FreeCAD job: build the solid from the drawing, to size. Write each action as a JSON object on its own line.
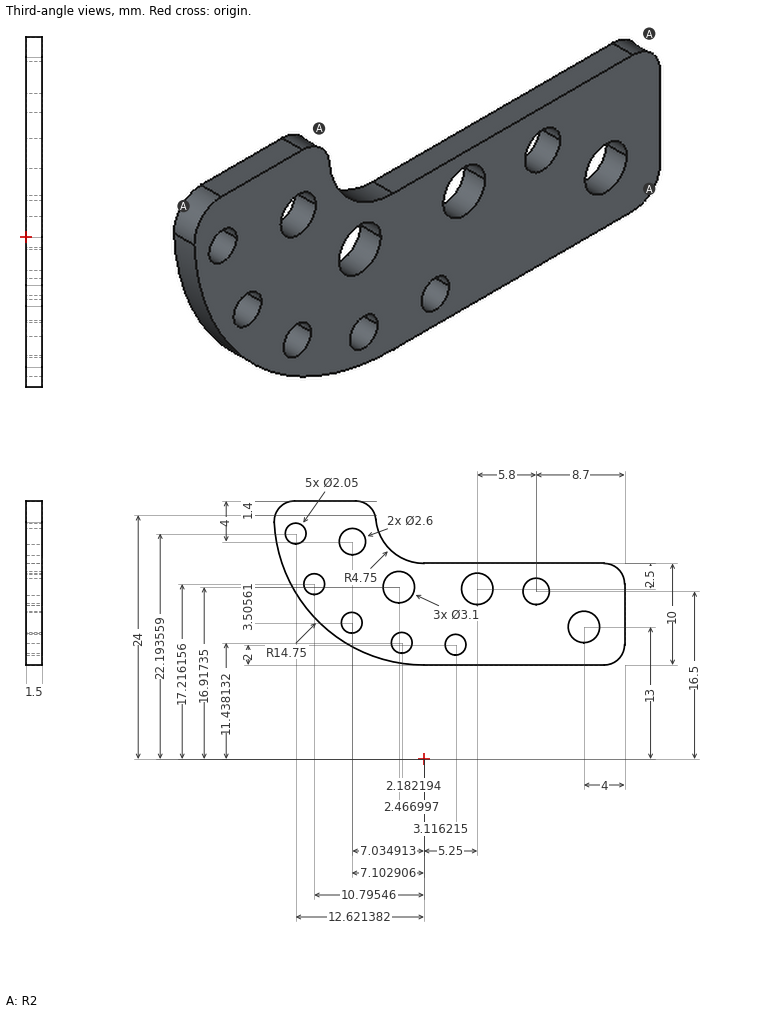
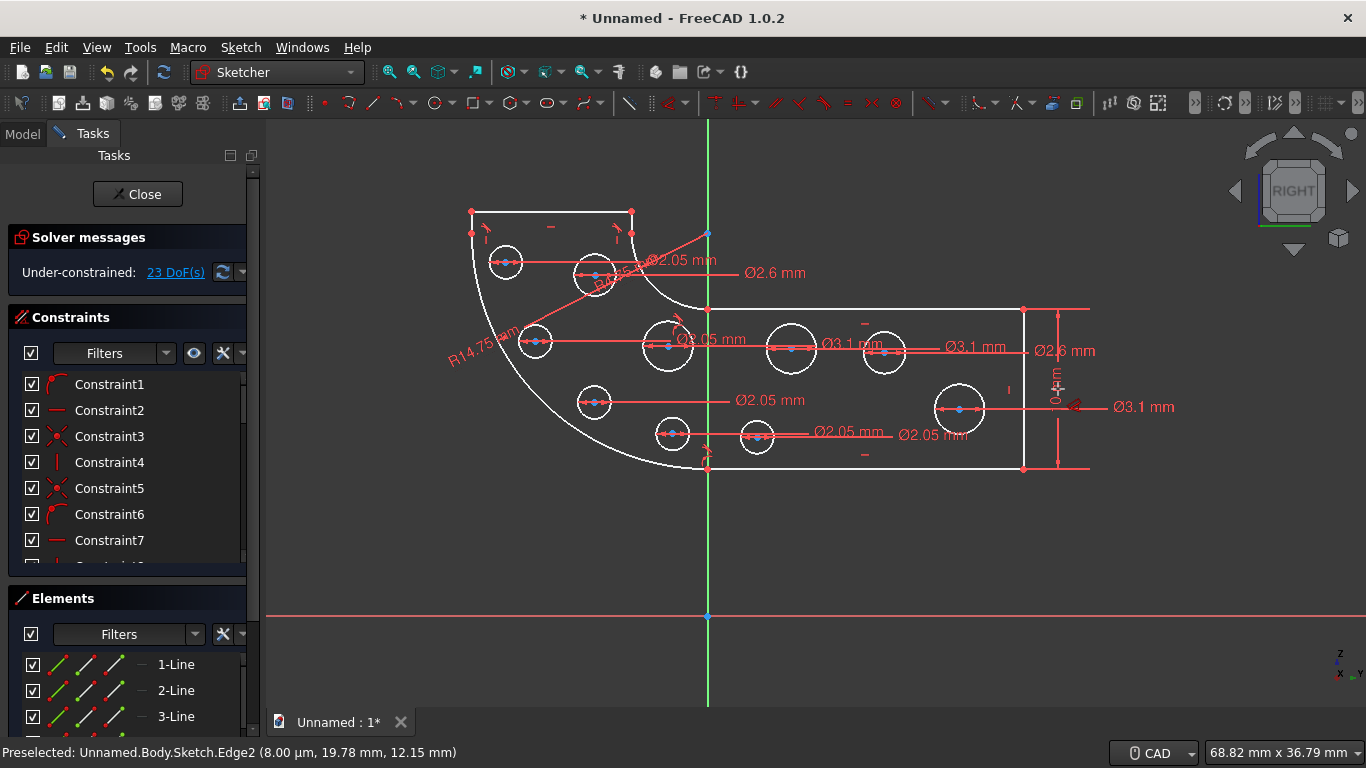
{"action": "left_click", "coordinate": [960, 409]}
{"action": "left_click", "coordinate": [994, 513]}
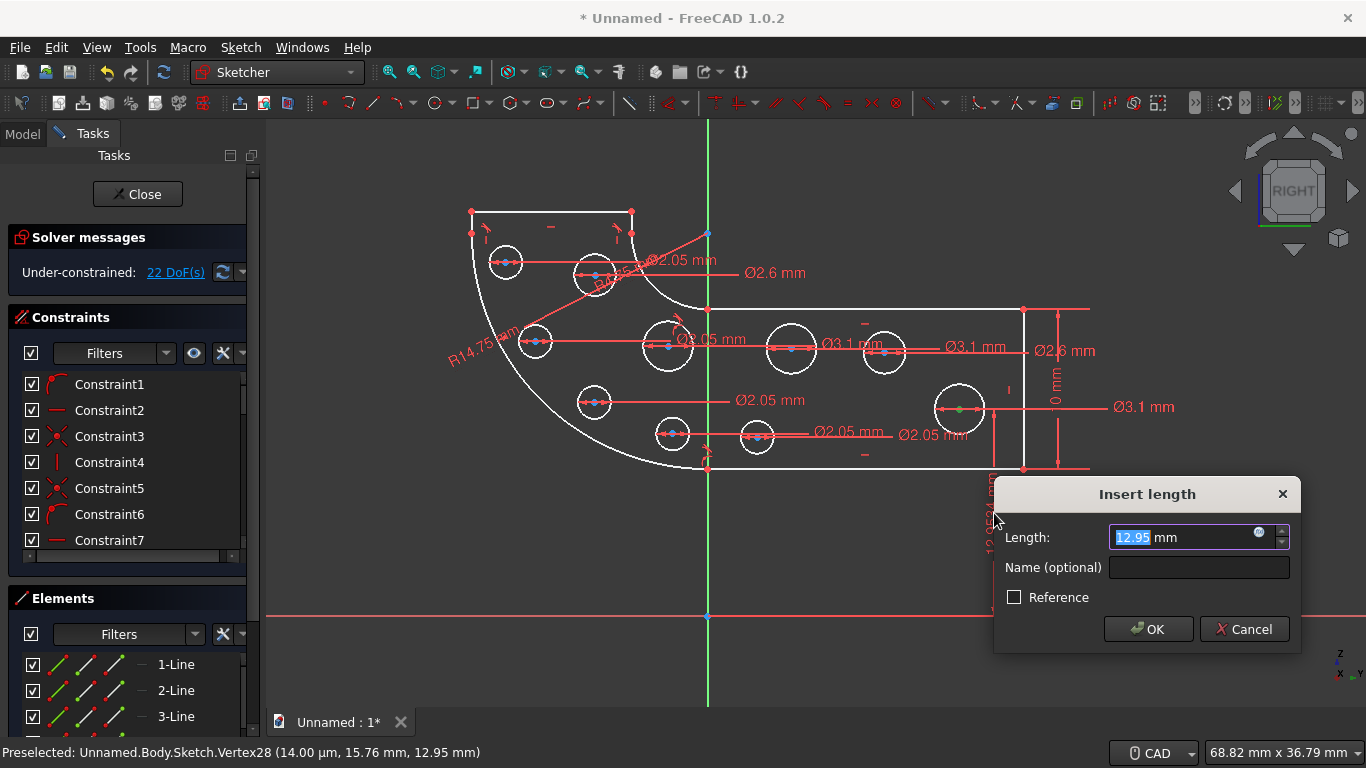
{"action": "type", "text": "13"}
{"action": "key", "text": "Return"}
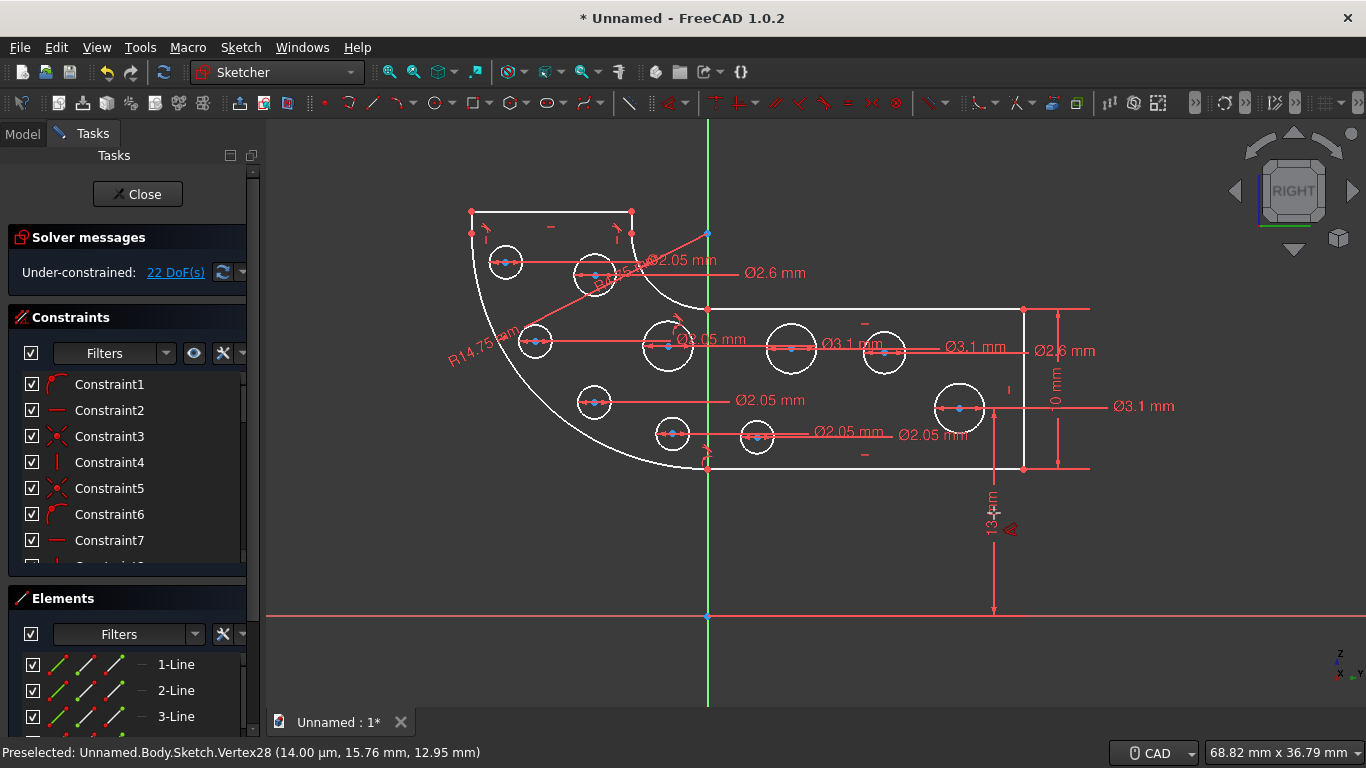
{"action": "left_click", "coordinate": [632, 212]}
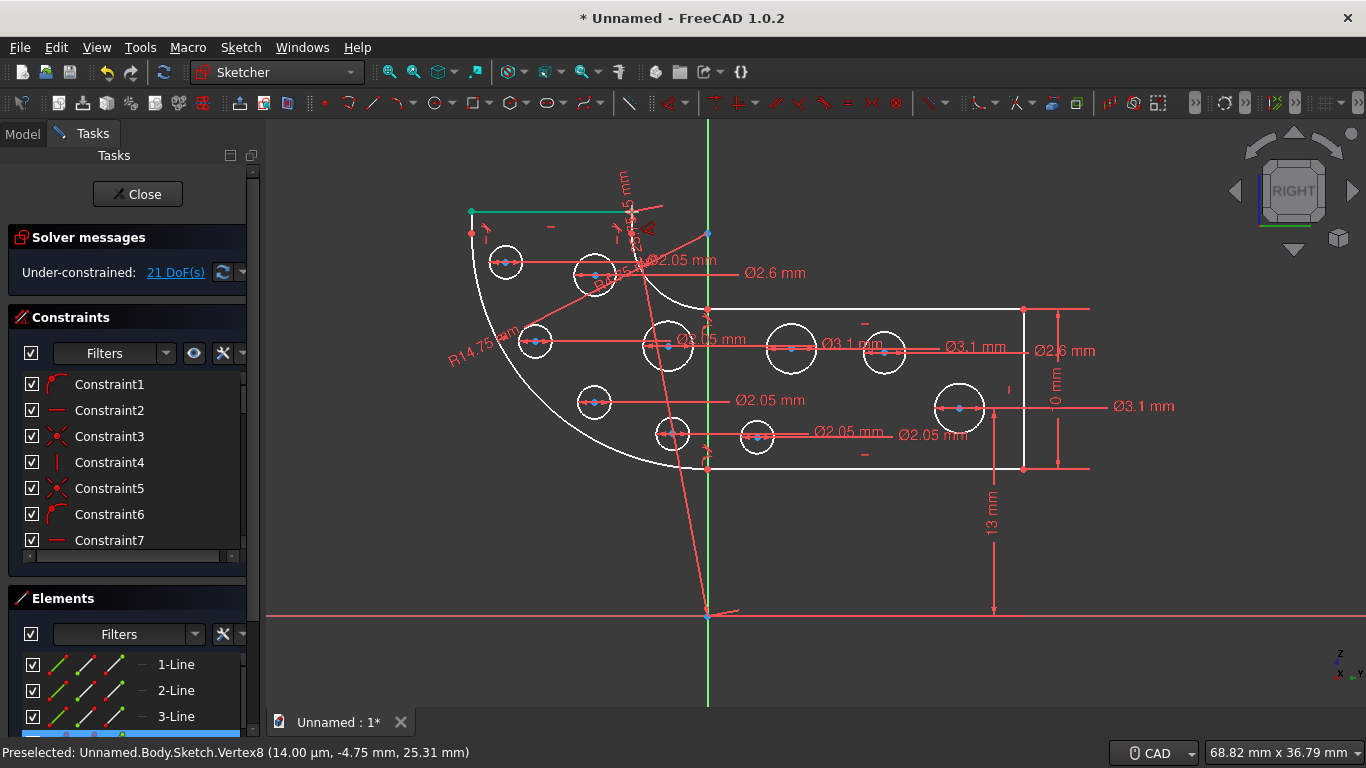
{"action": "left_click", "coordinate": [595, 275]}
{"action": "left_click", "coordinate": [561, 243]}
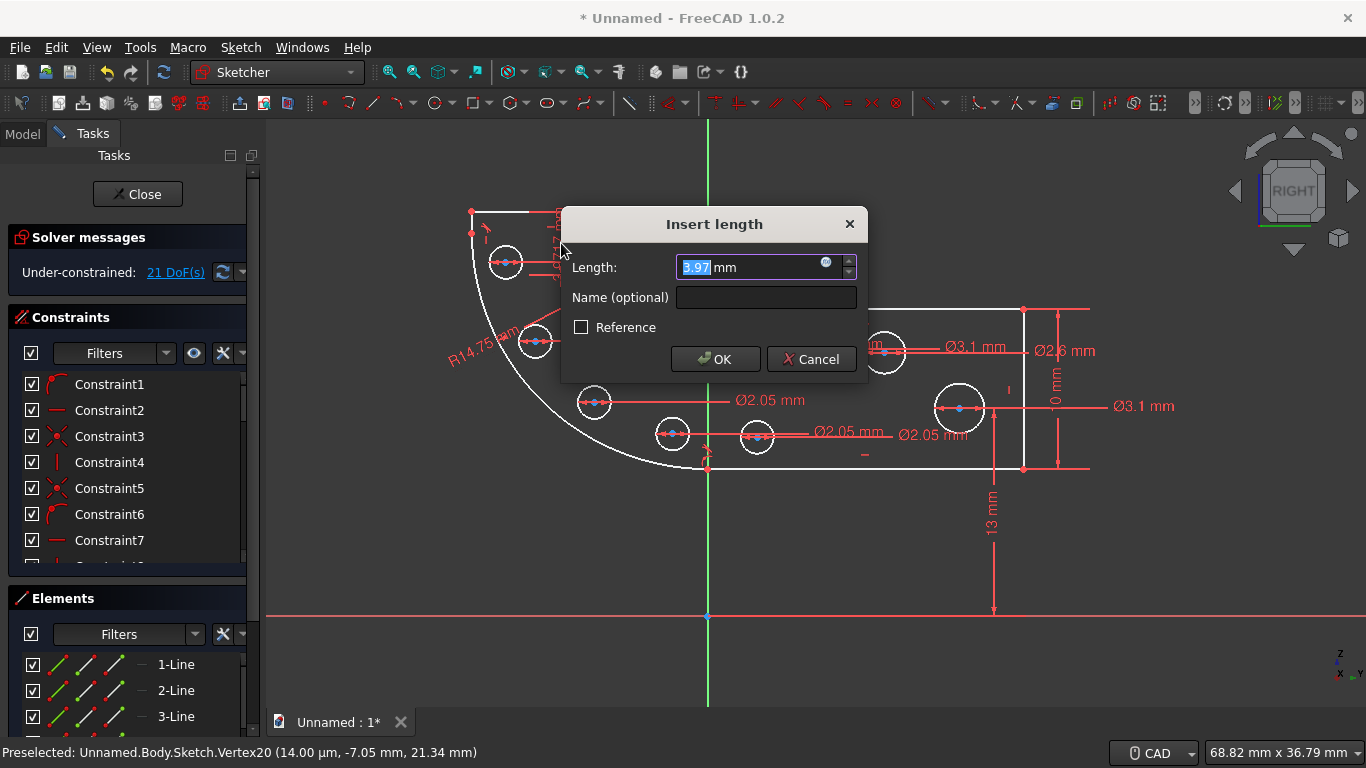
{"action": "type", "text": "4"}
{"action": "key", "text": "Return"}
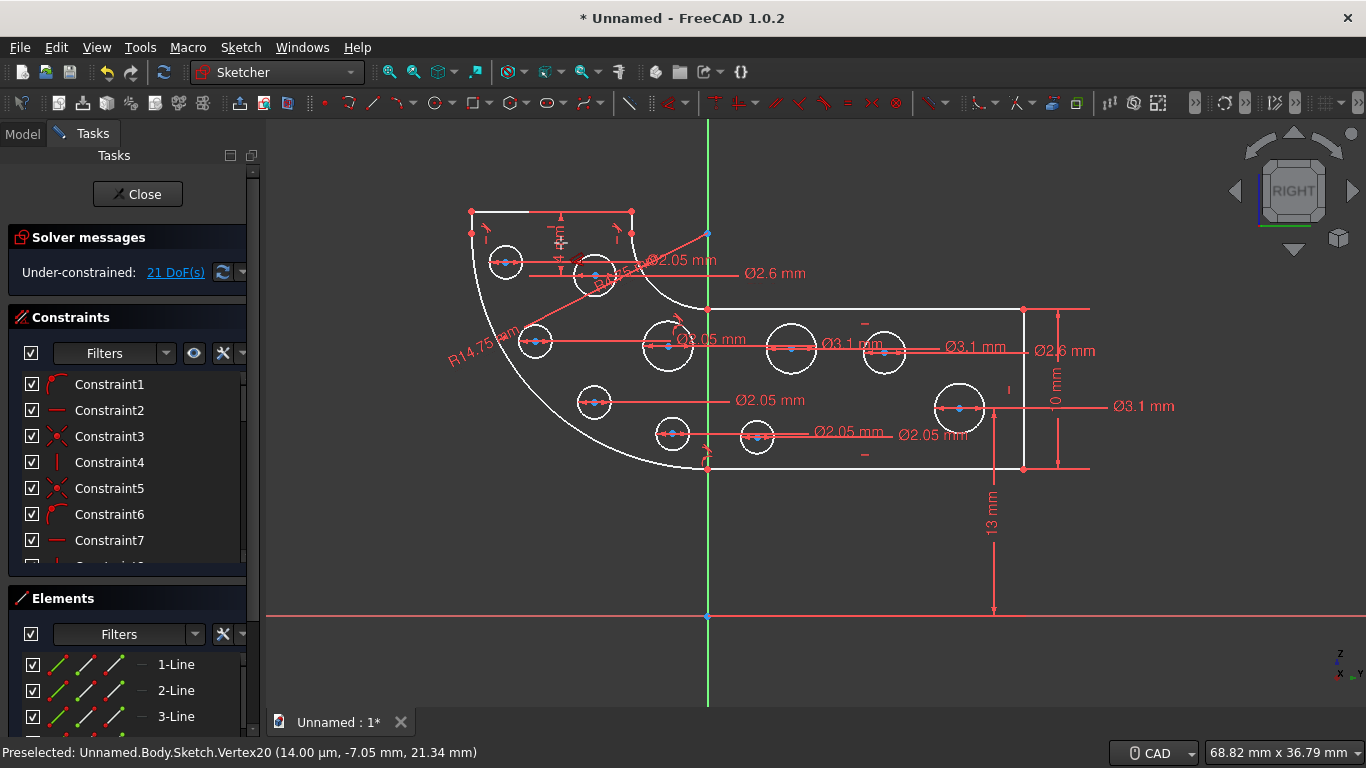
{"action": "scroll", "coordinate": [708, 469], "scroll_direction": "up", "scroll_amount": 2}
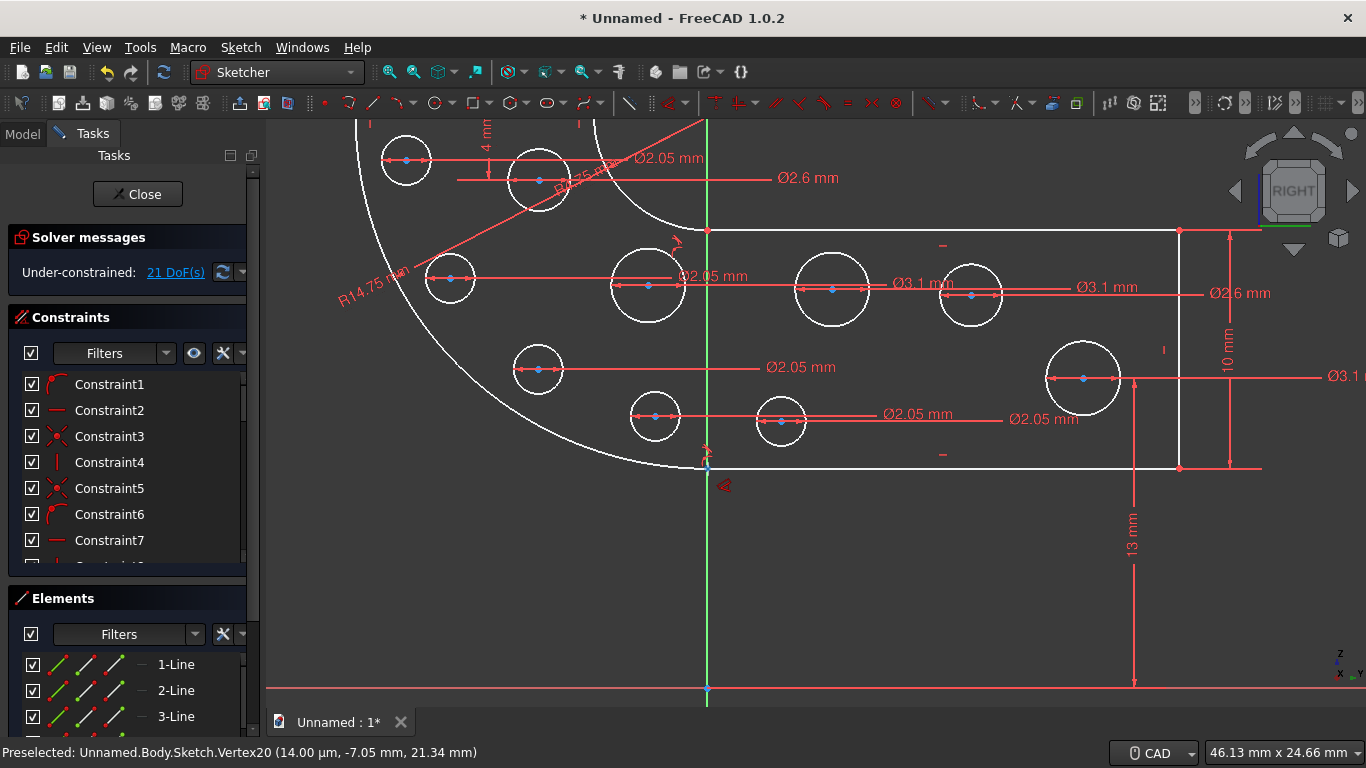
{"action": "left_click", "coordinate": [707, 469]}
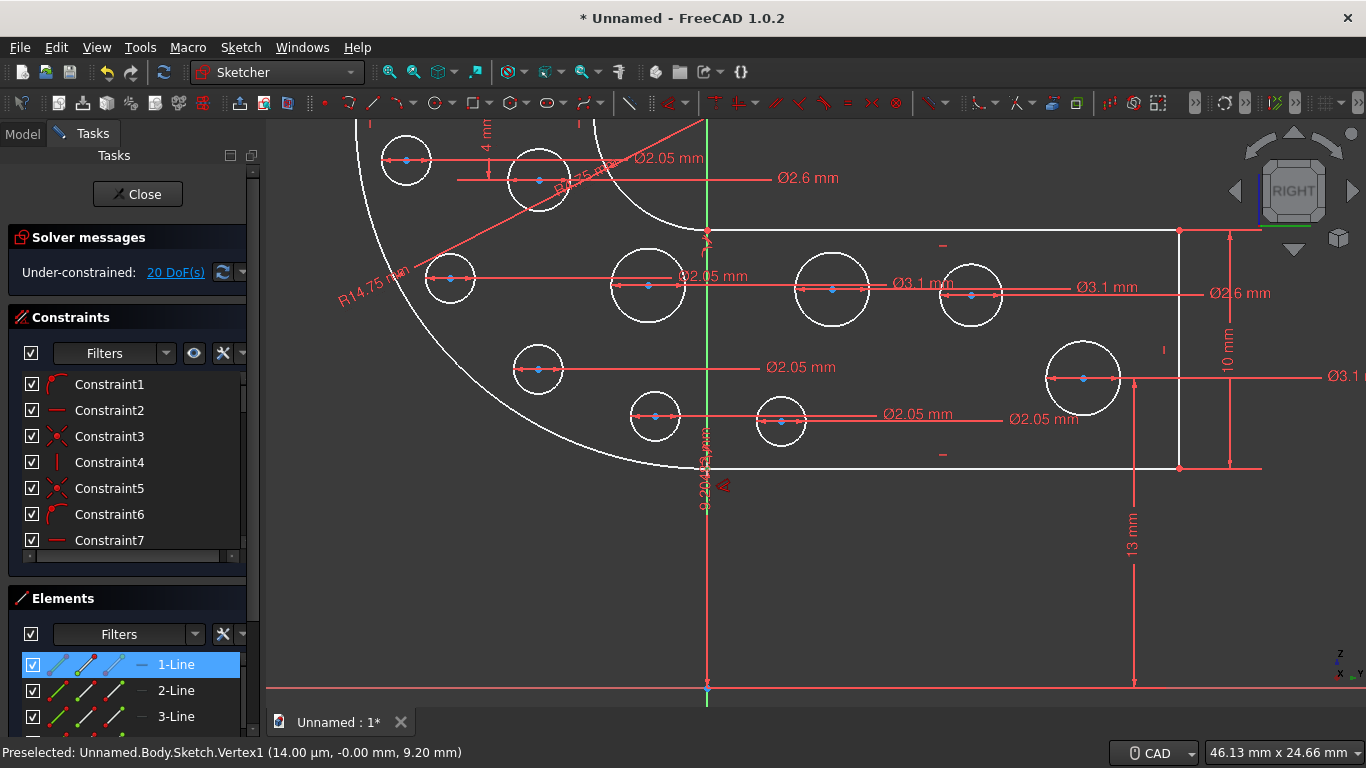
{"action": "left_click", "coordinate": [781, 421]}
{"action": "left_click", "coordinate": [815, 445]}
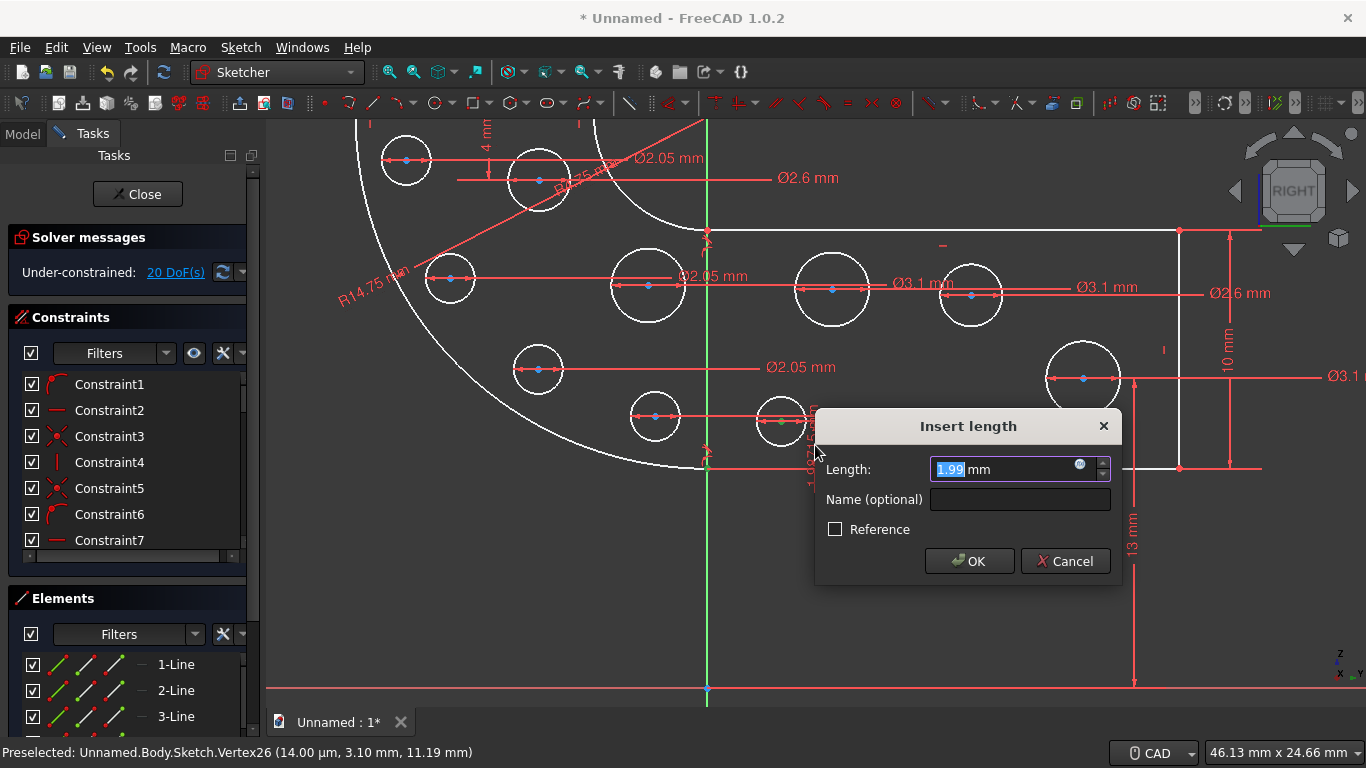
{"action": "type", "text": "2"}
{"action": "key", "text": "Return"}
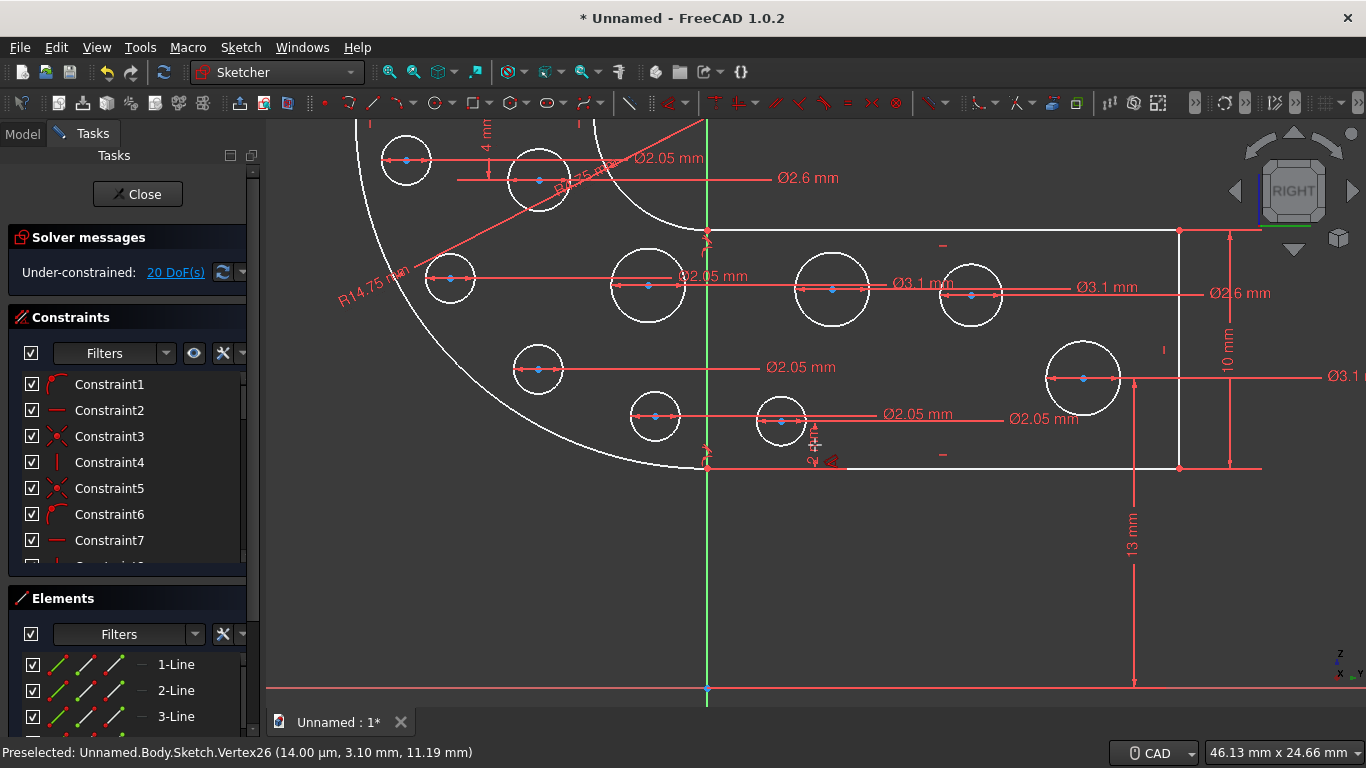
{"action": "left_click", "coordinate": [1179, 469]}